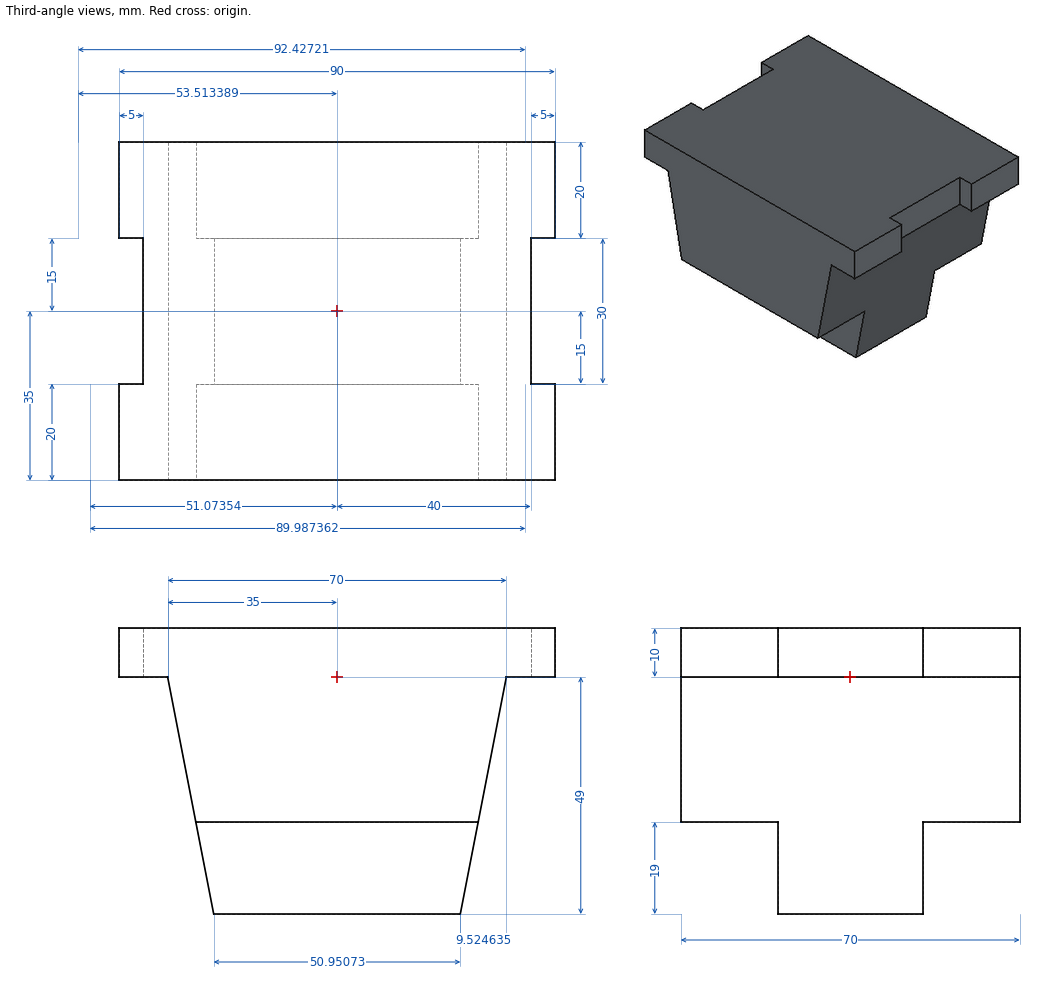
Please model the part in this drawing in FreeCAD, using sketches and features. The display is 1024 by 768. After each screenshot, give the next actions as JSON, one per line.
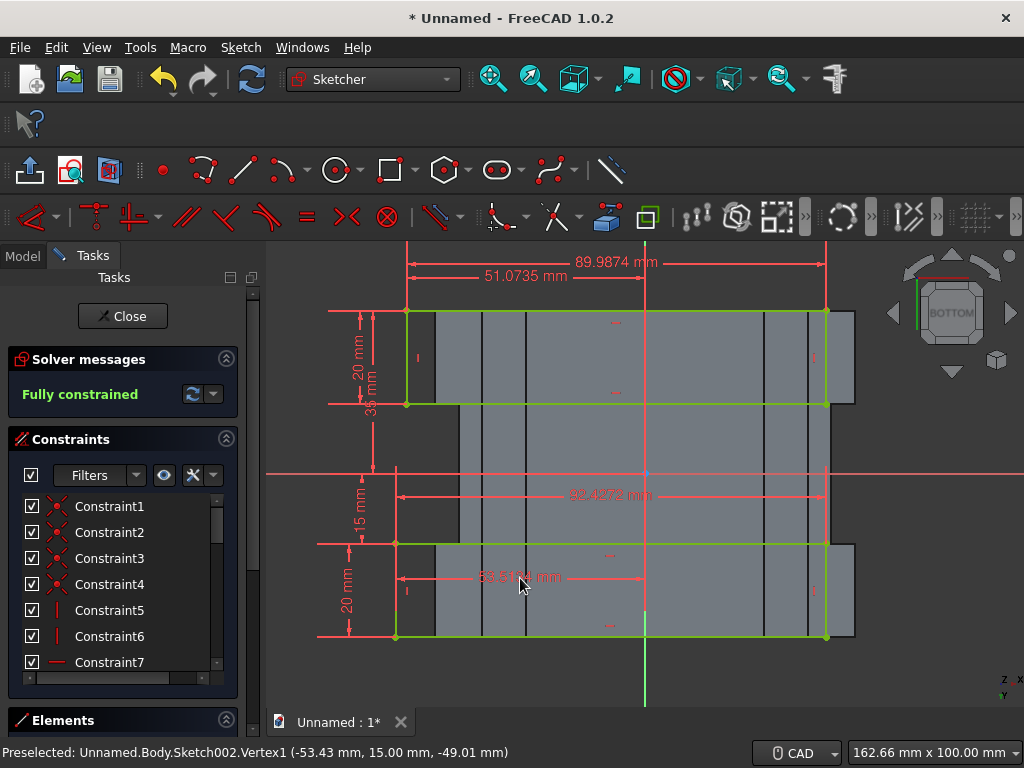
{"action": "left_click", "coordinate": [123, 316]}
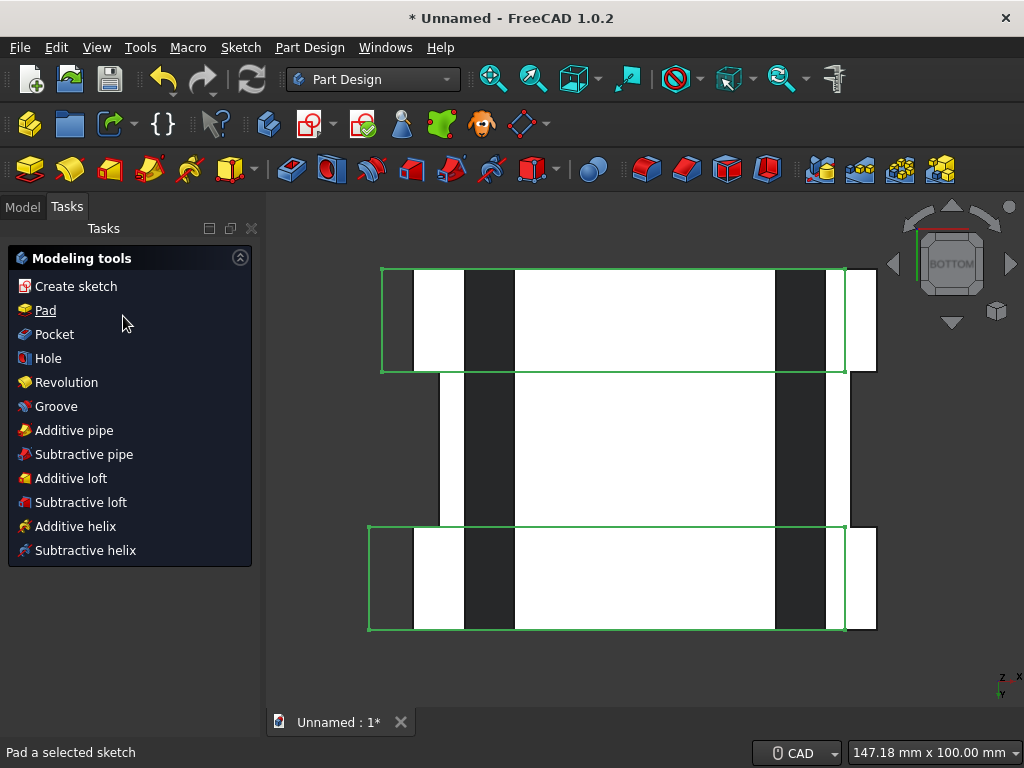
{"action": "left_click", "coordinate": [292, 170]}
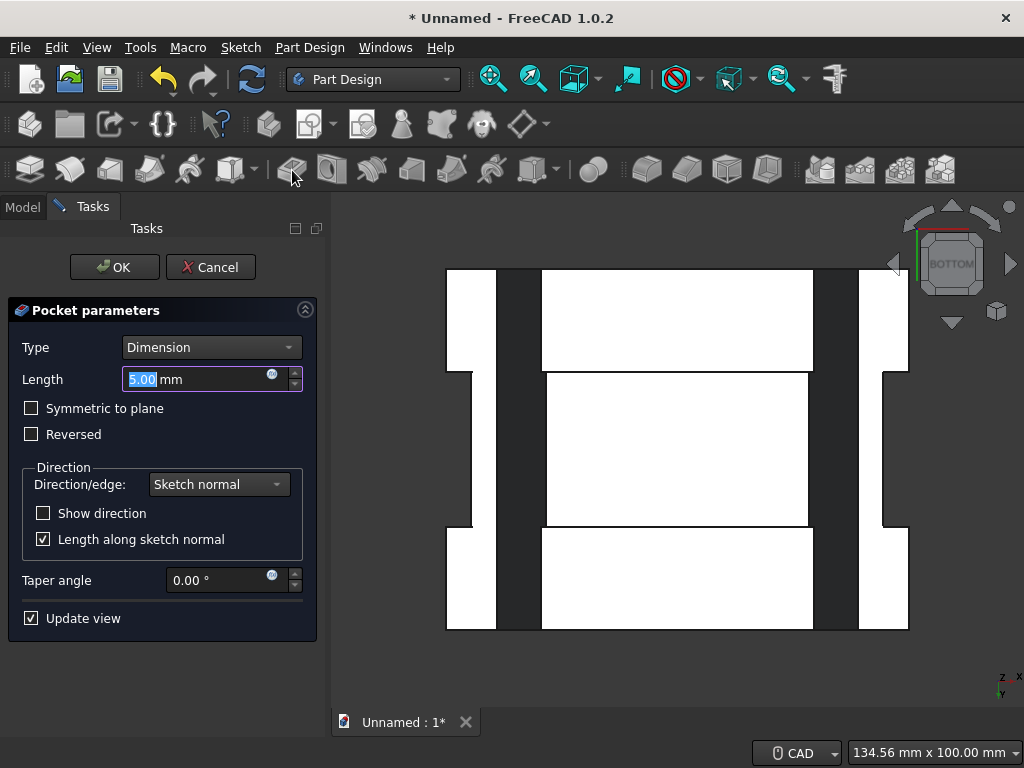
{"action": "type", "text": "19"}
{"action": "key", "text": "Tab"}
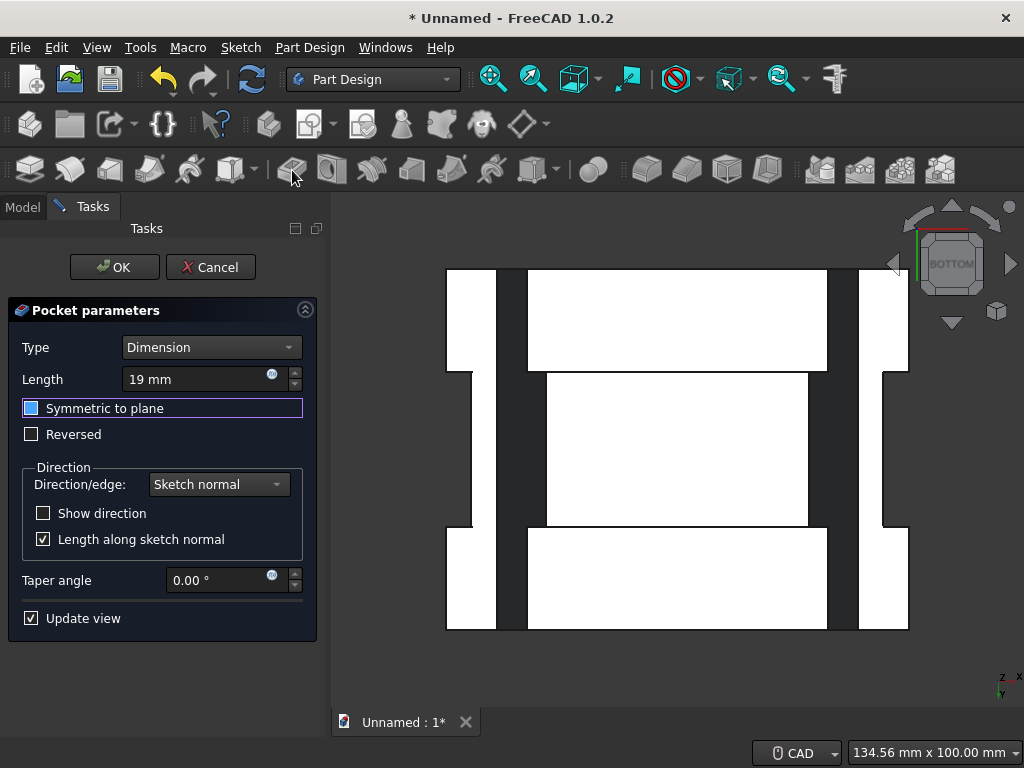
{"action": "left_click", "coordinate": [115, 267]}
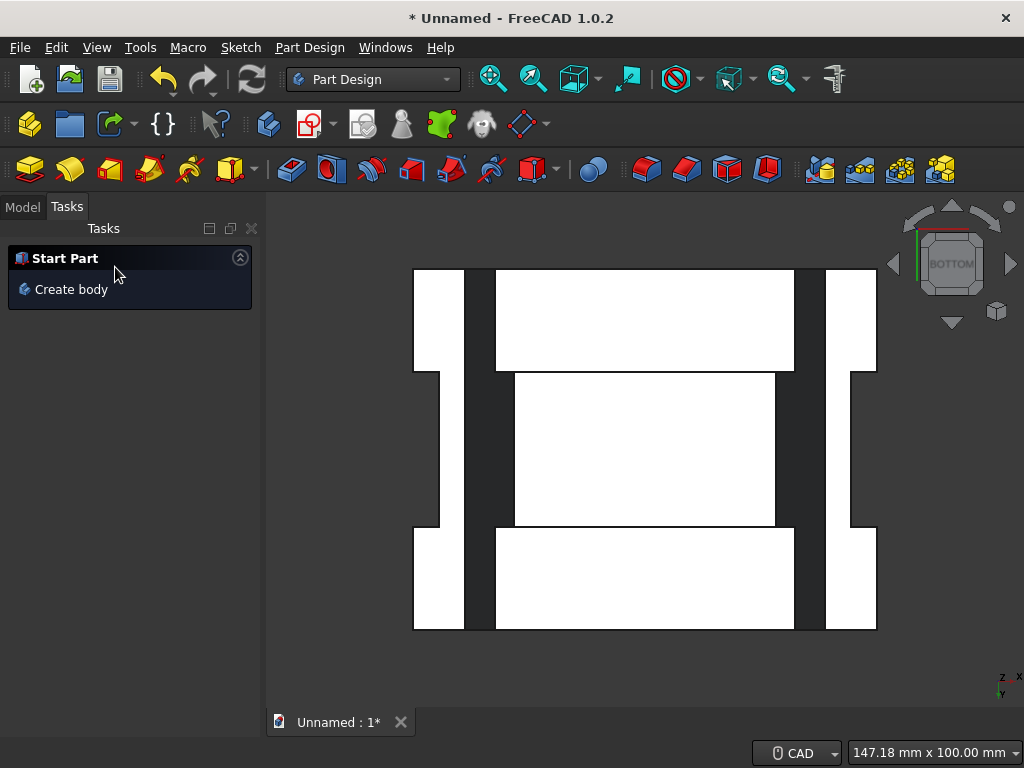
{"action": "key", "text": "0"}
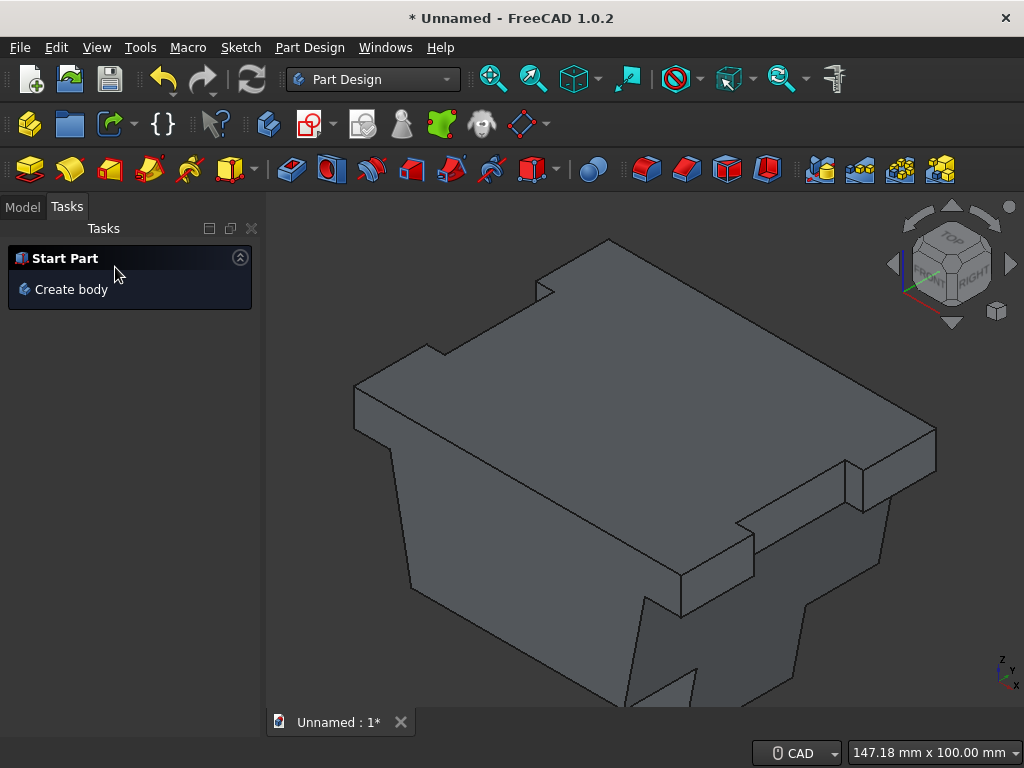
{"action": "key", "text": "v f"}